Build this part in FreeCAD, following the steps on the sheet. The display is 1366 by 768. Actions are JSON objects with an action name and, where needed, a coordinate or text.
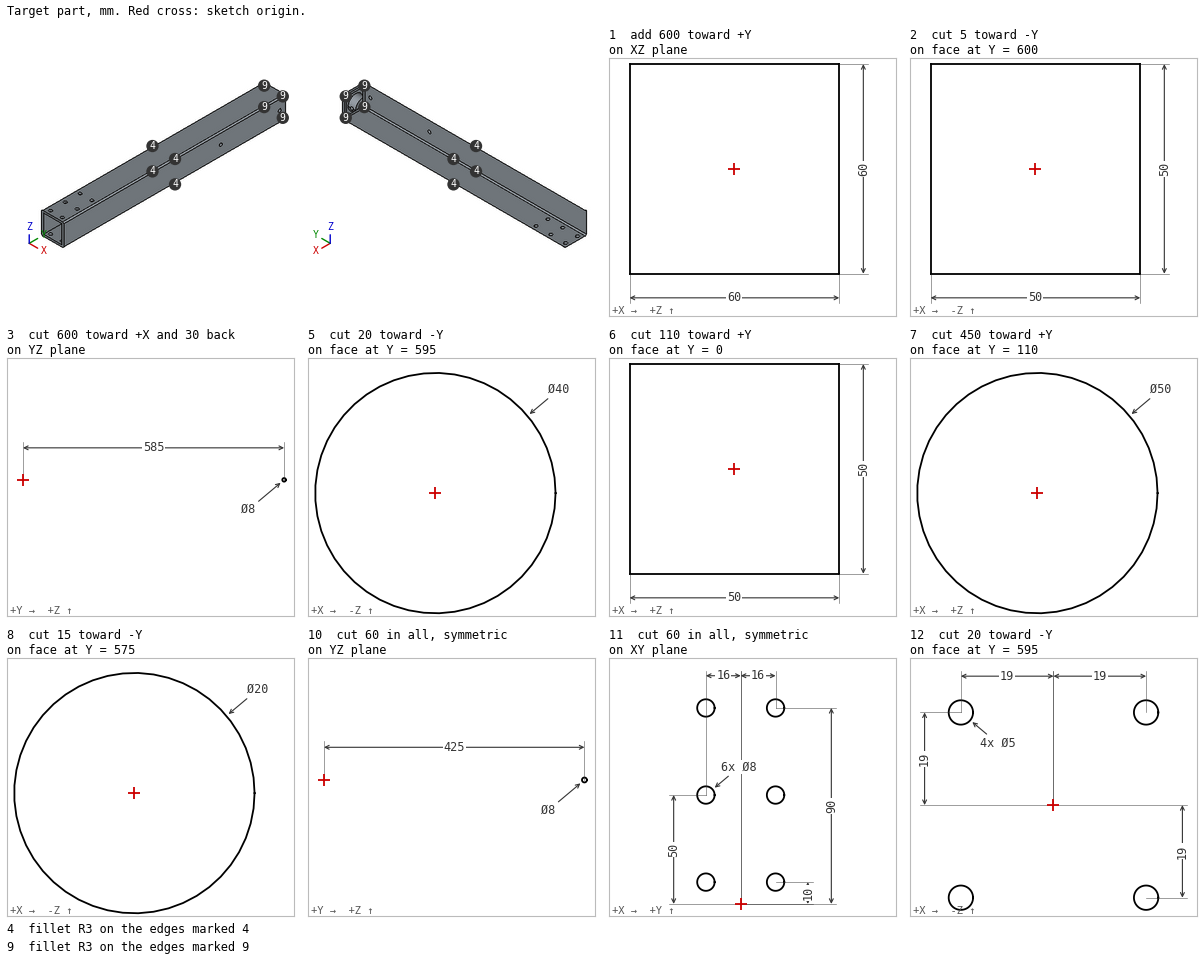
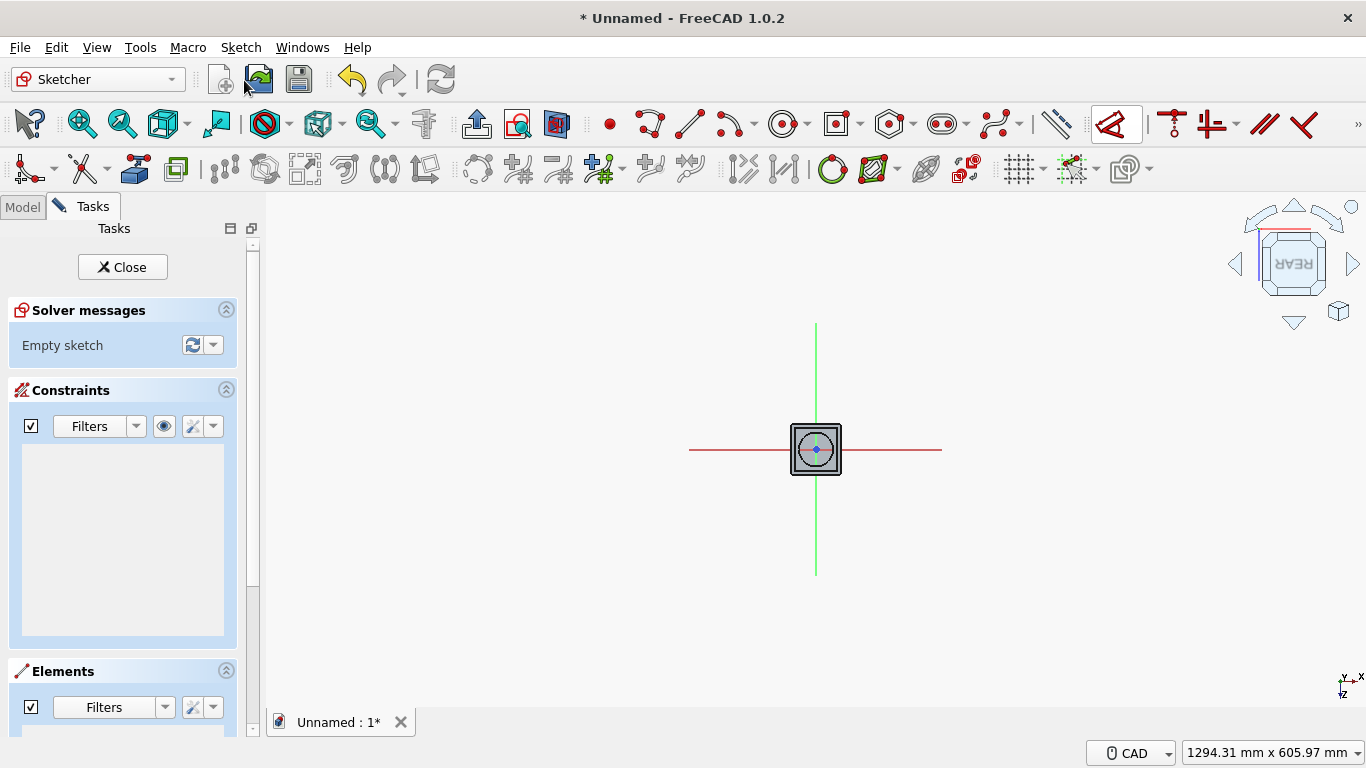
{"action": "scroll", "coordinate": [820, 449], "scroll_direction": "up", "scroll_amount": 15}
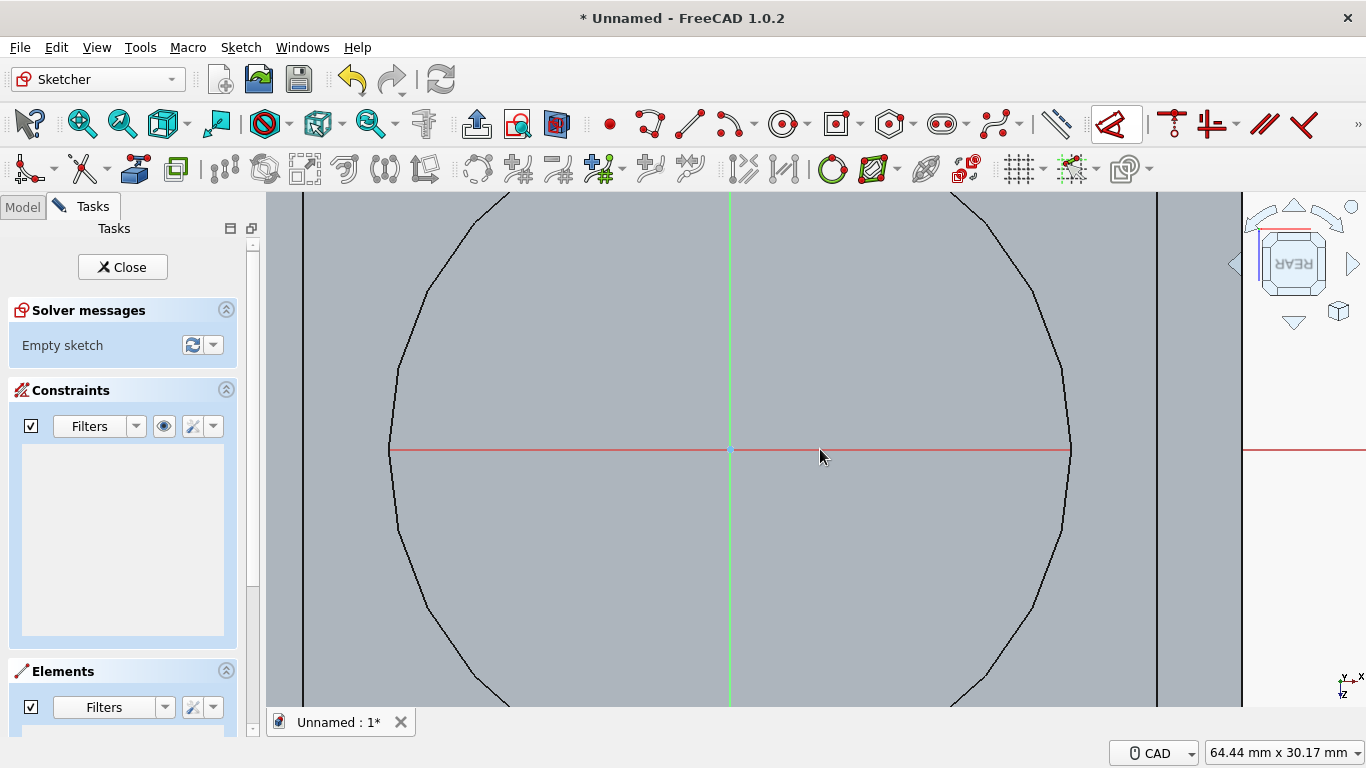
{"action": "left_click", "coordinate": [784, 124]}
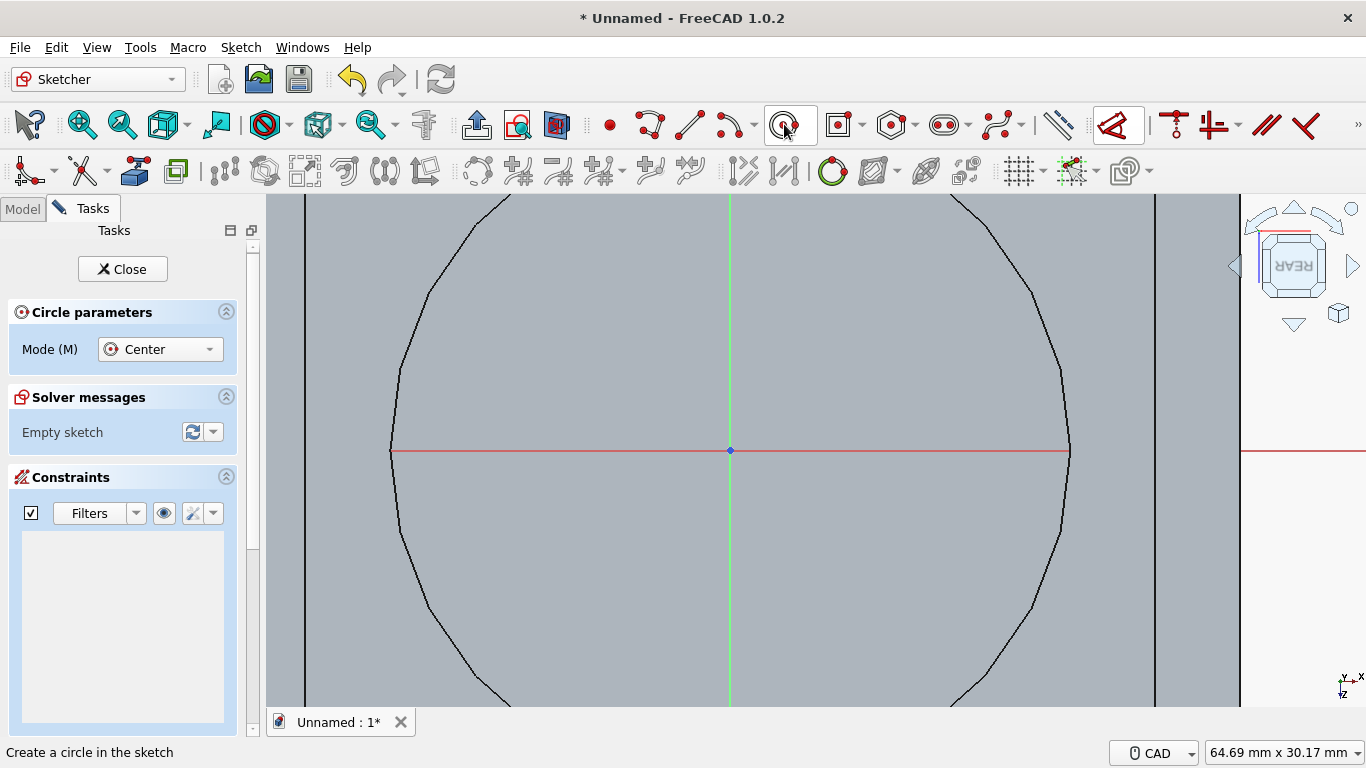
{"action": "left_click", "coordinate": [730, 450]}
{"action": "mouse_move", "coordinate": [851, 330]}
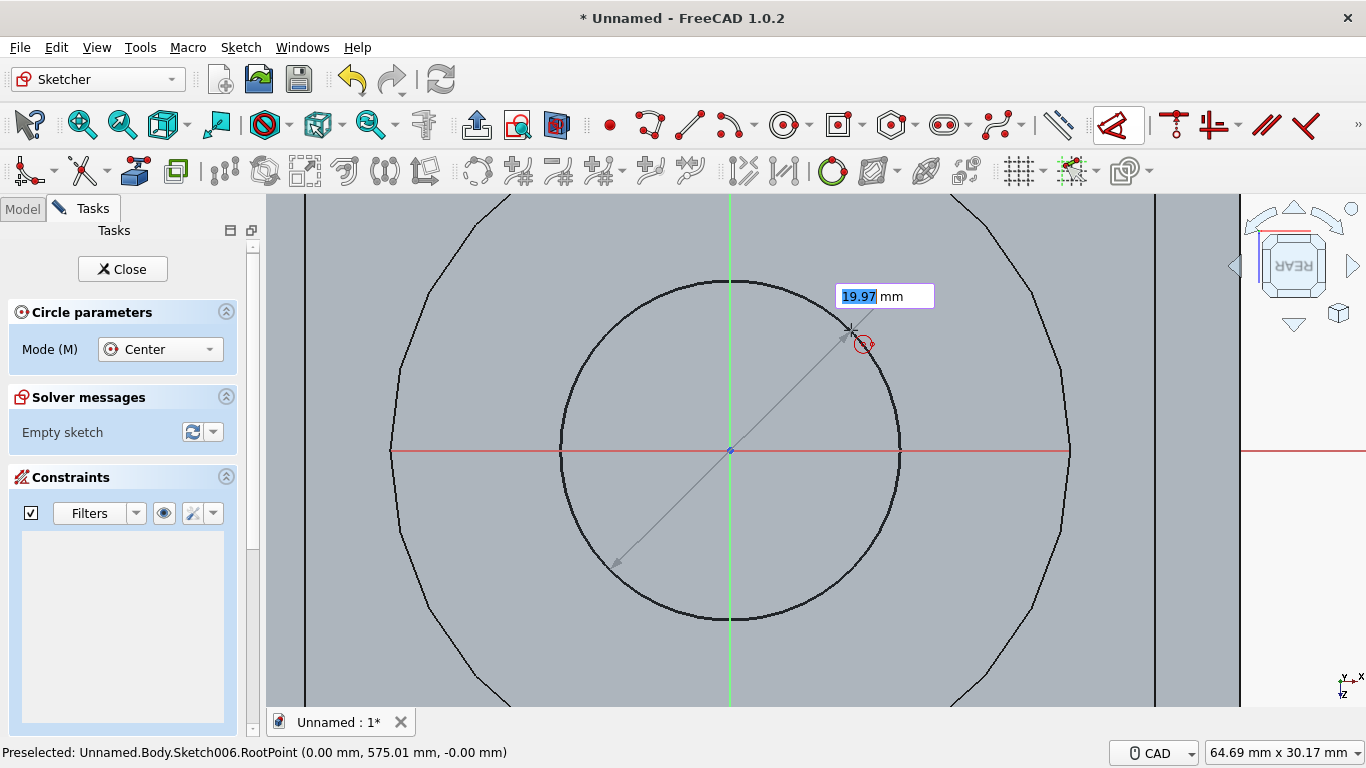
{"action": "type", "text": "20"}
{"action": "key", "text": "Return"}
{"action": "key", "text": "Escape"}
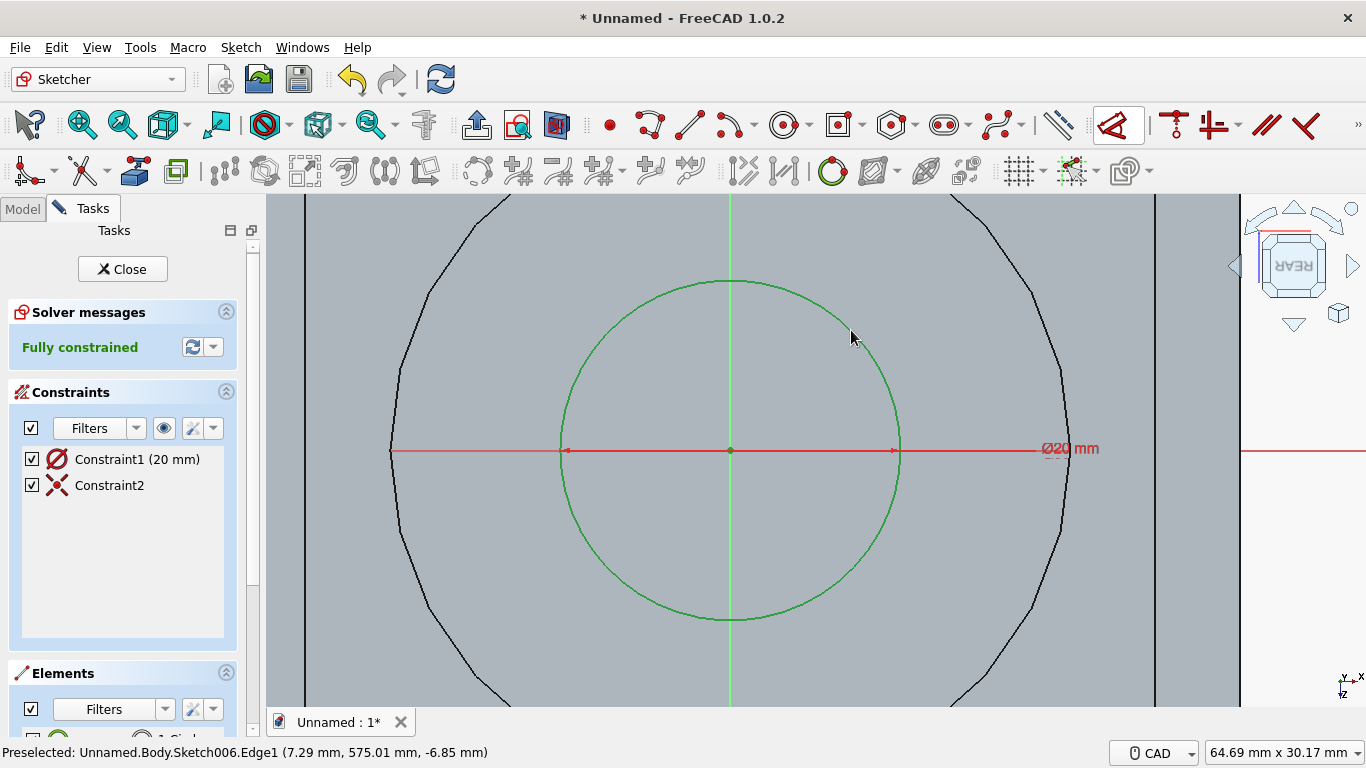
{"action": "left_click", "coordinate": [123, 269]}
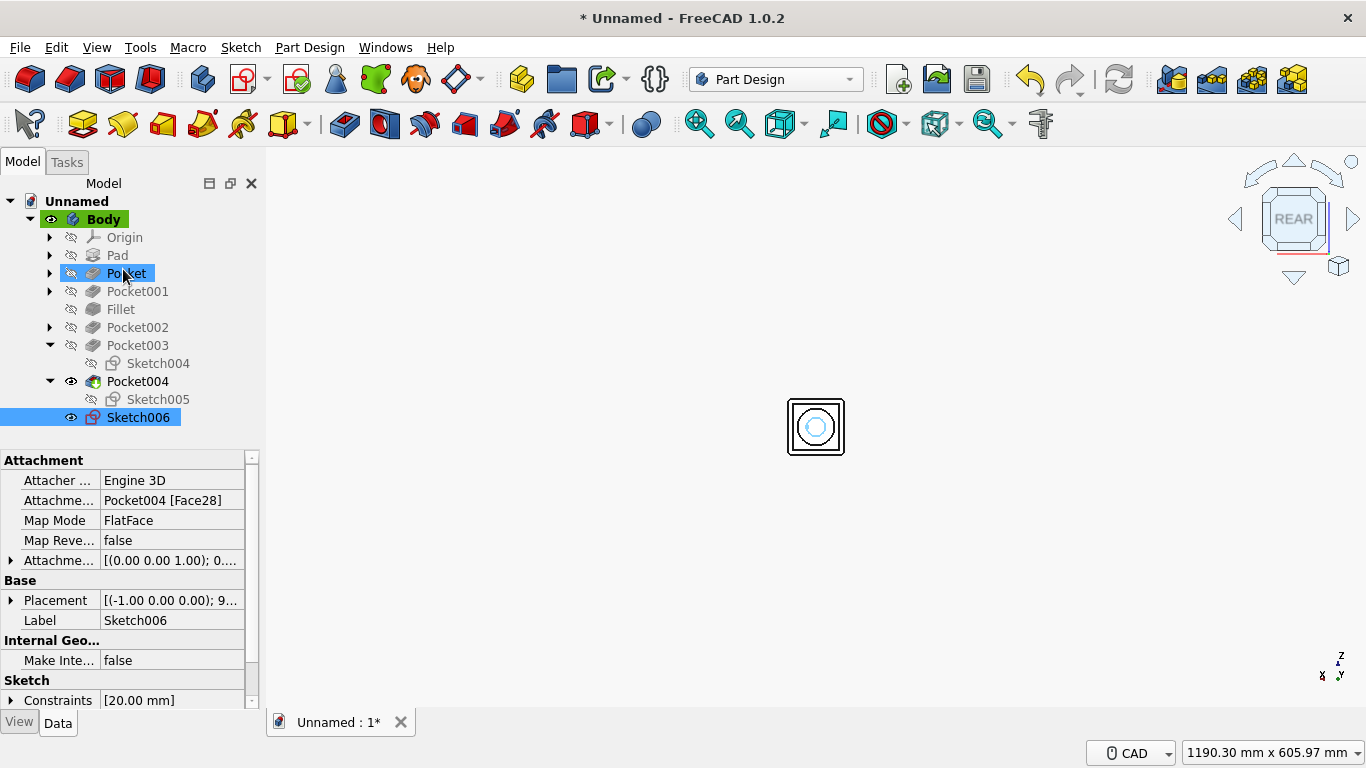
{"action": "left_click", "coordinate": [346, 124]}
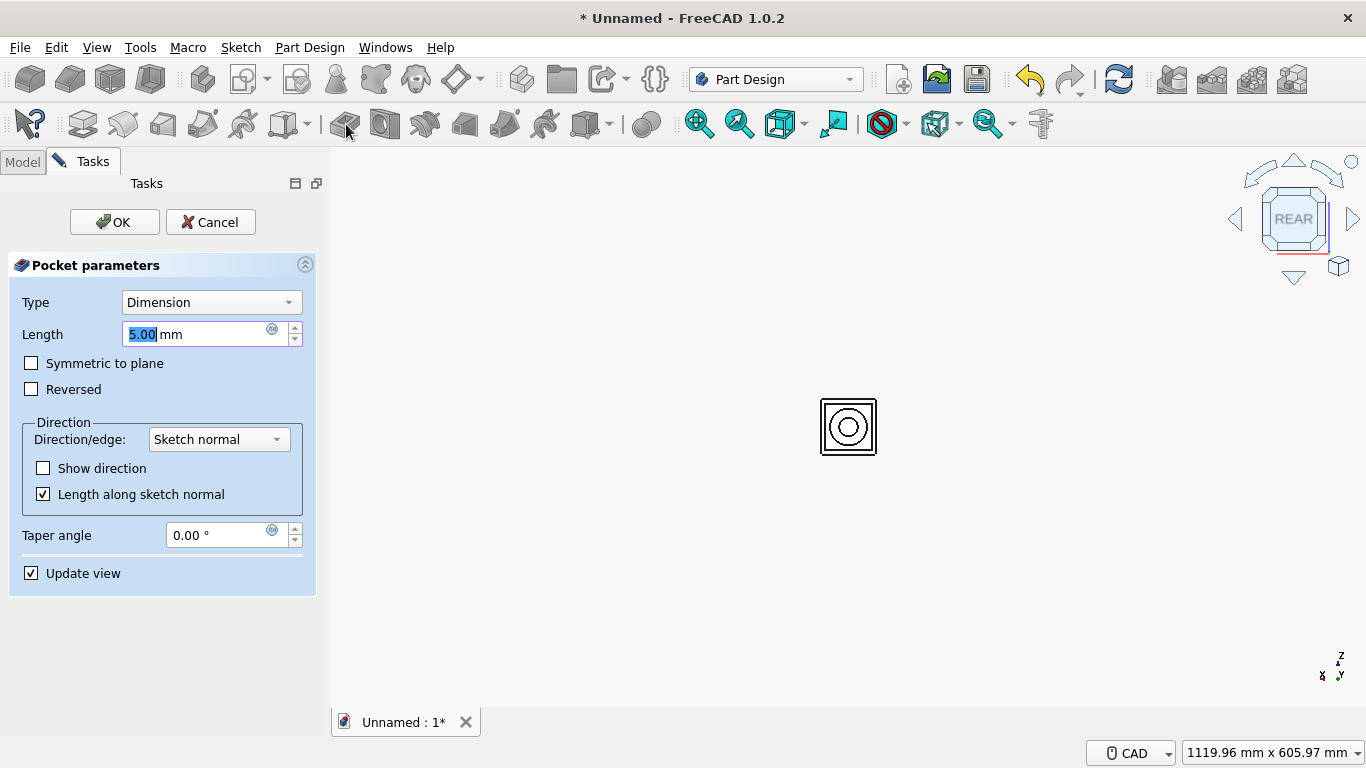
{"action": "type", "text": "15"}
{"action": "key", "text": "Tab"}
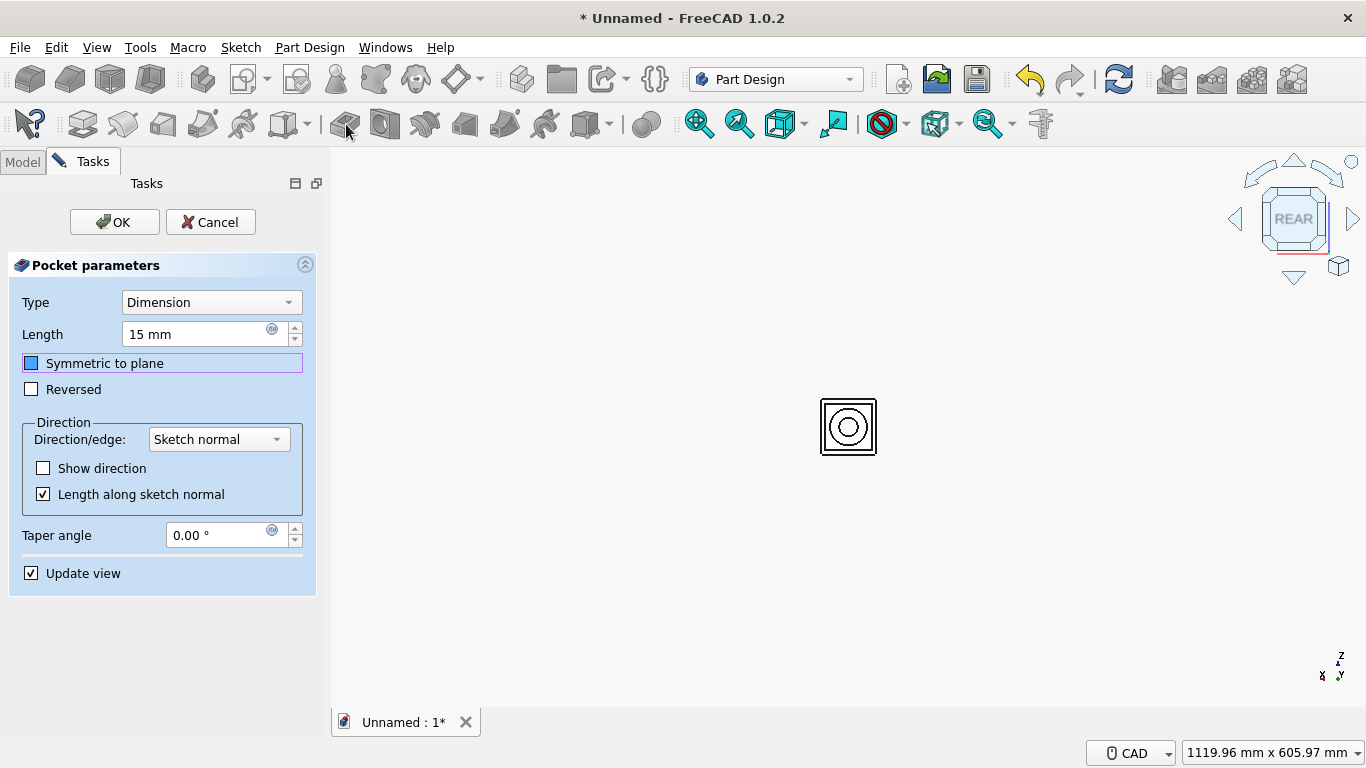
{"action": "left_click", "coordinate": [115, 222]}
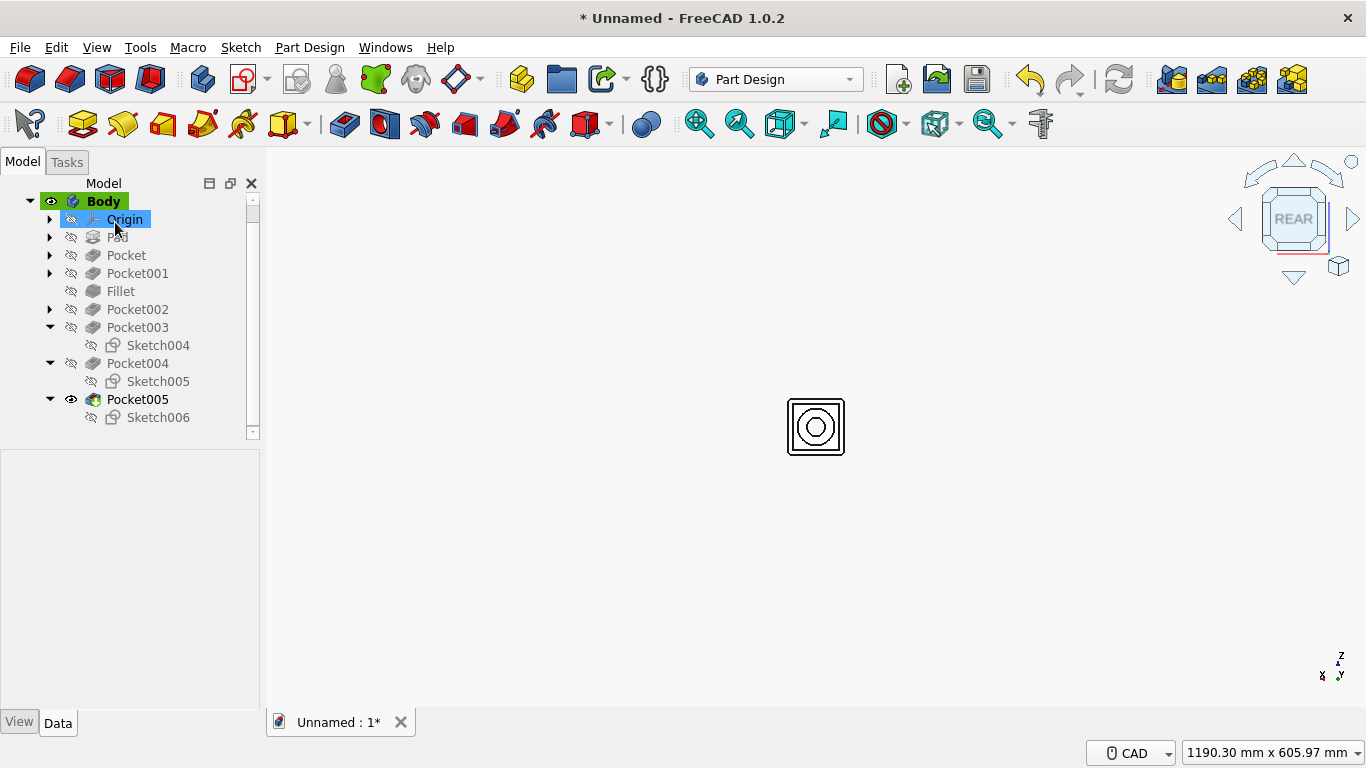
{"action": "key", "text": "v f"}